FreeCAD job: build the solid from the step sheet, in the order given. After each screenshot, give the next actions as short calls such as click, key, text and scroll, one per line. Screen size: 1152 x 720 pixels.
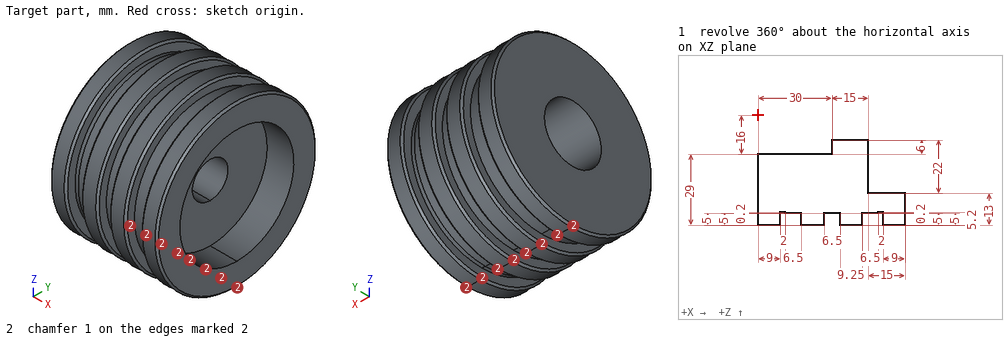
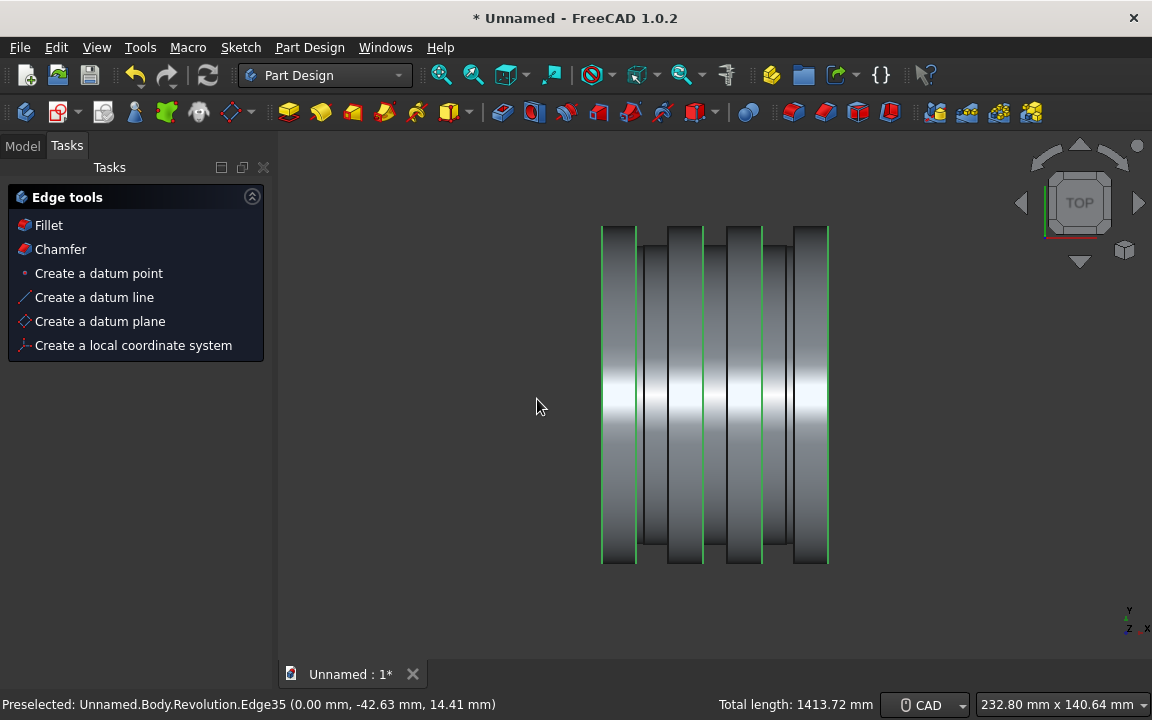
click(794, 394, ctrl)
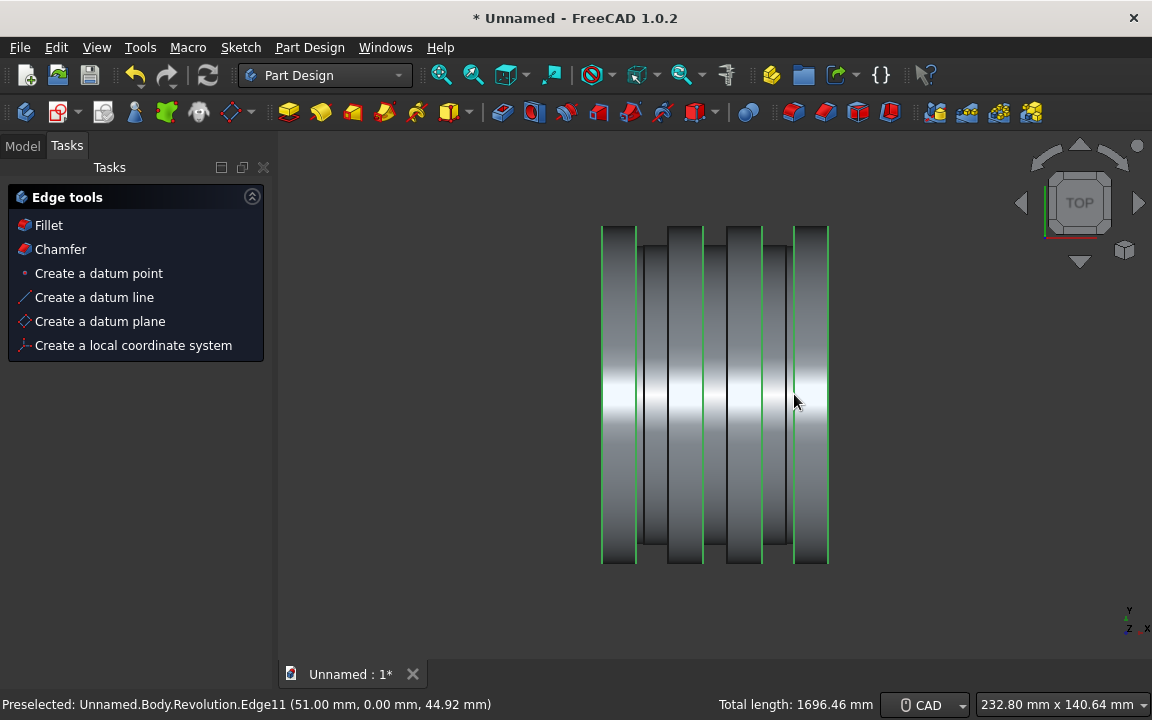
click(727, 394, ctrl)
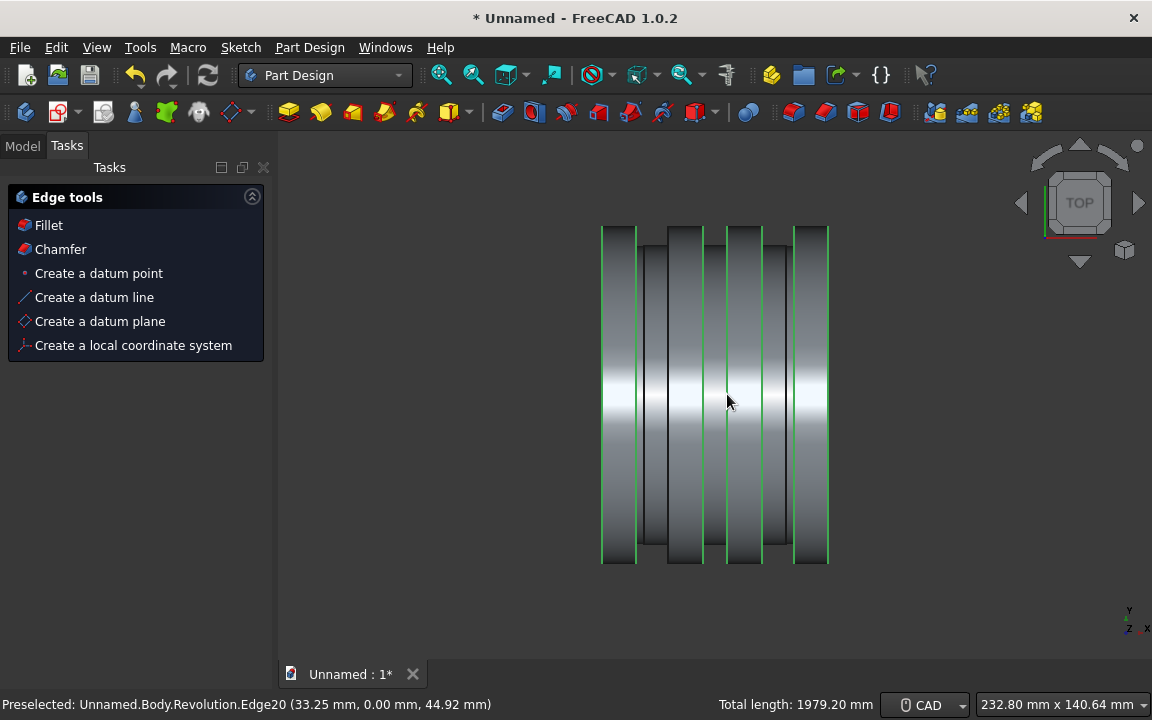
click(668, 394, ctrl)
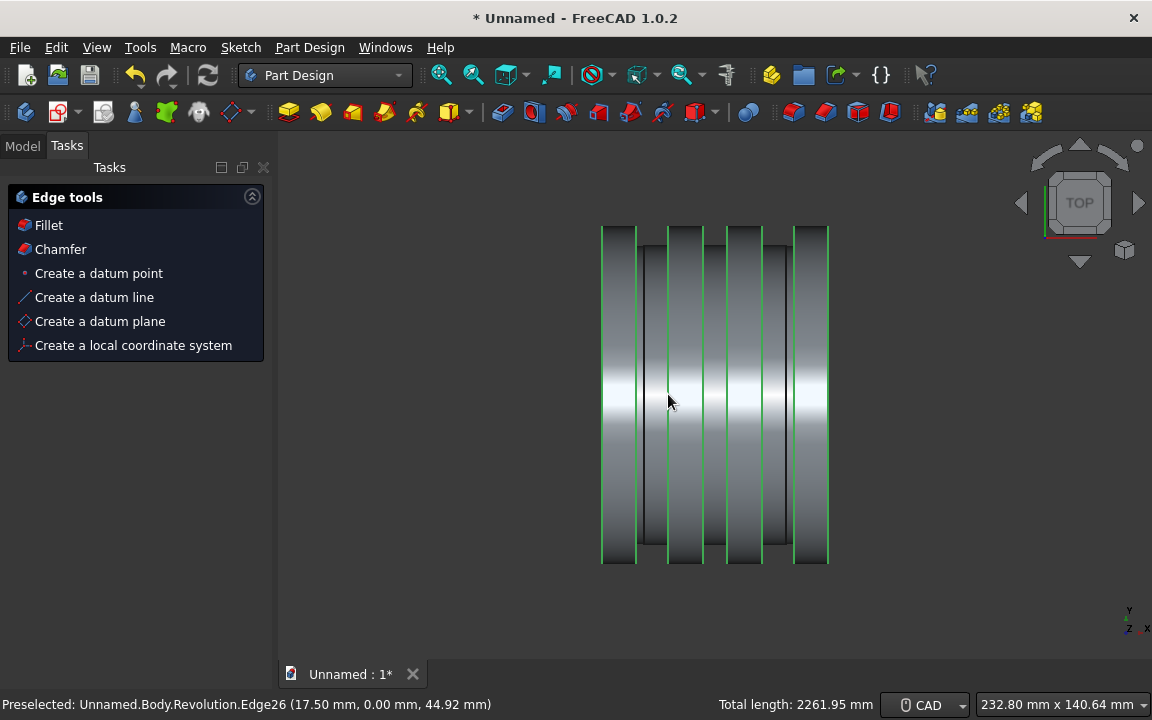
click(826, 112)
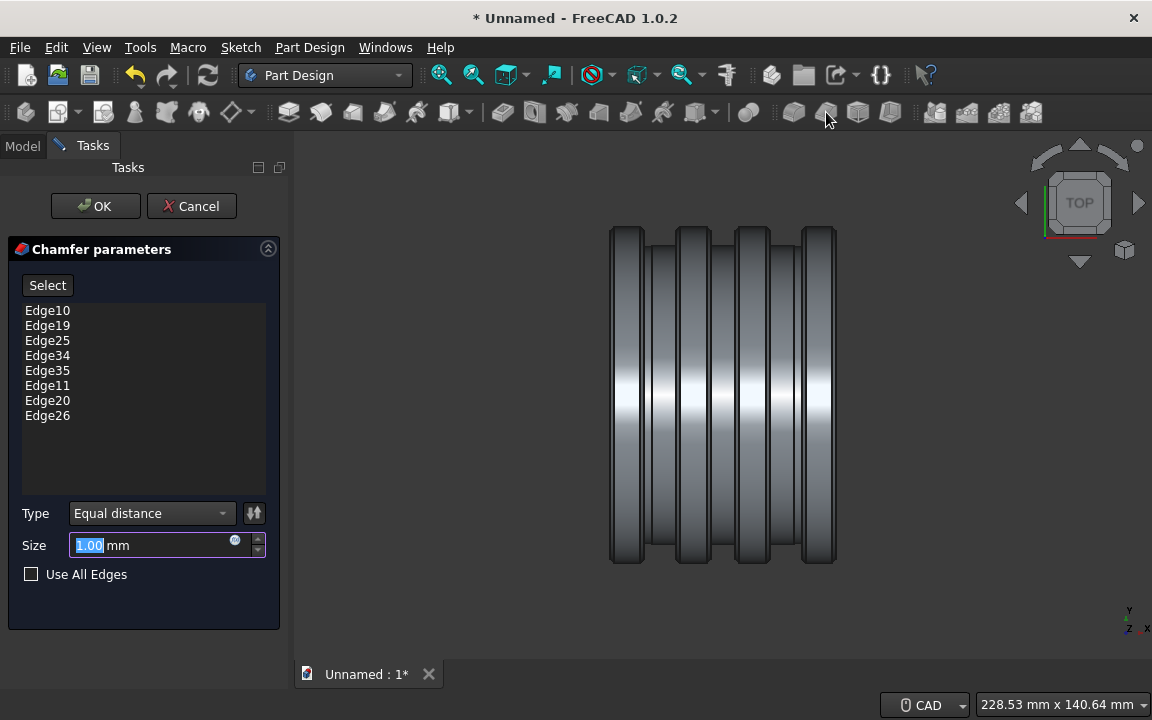
text(1)
key(Tab)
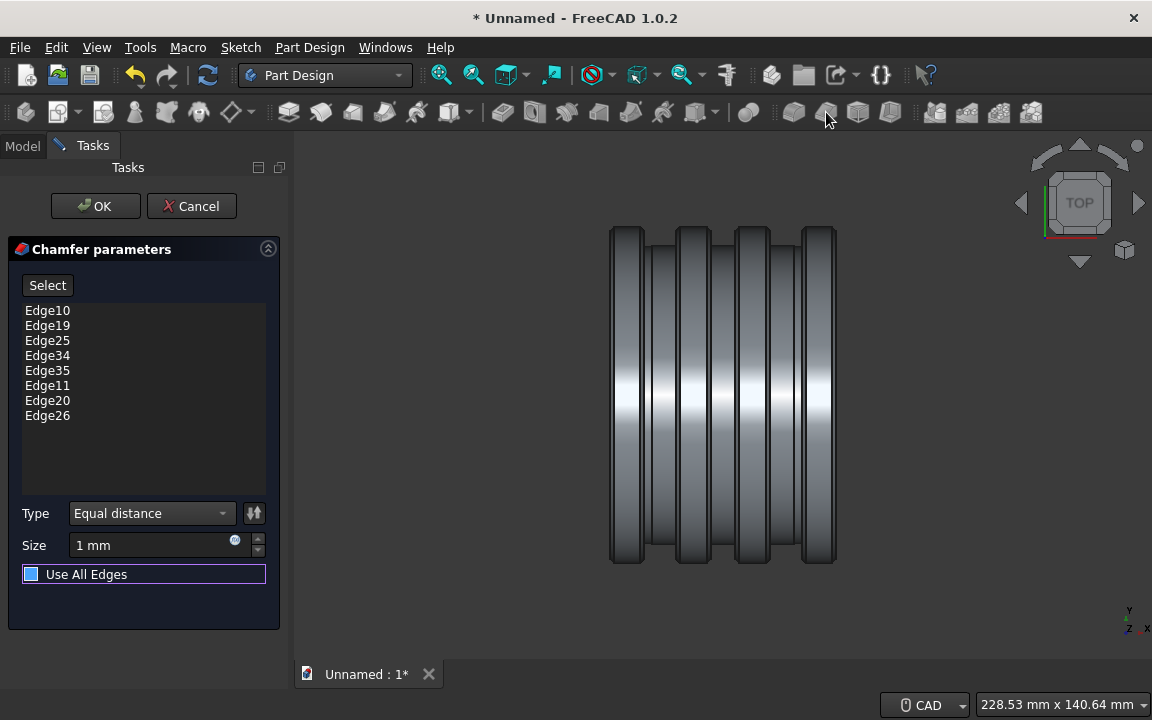
click(96, 206)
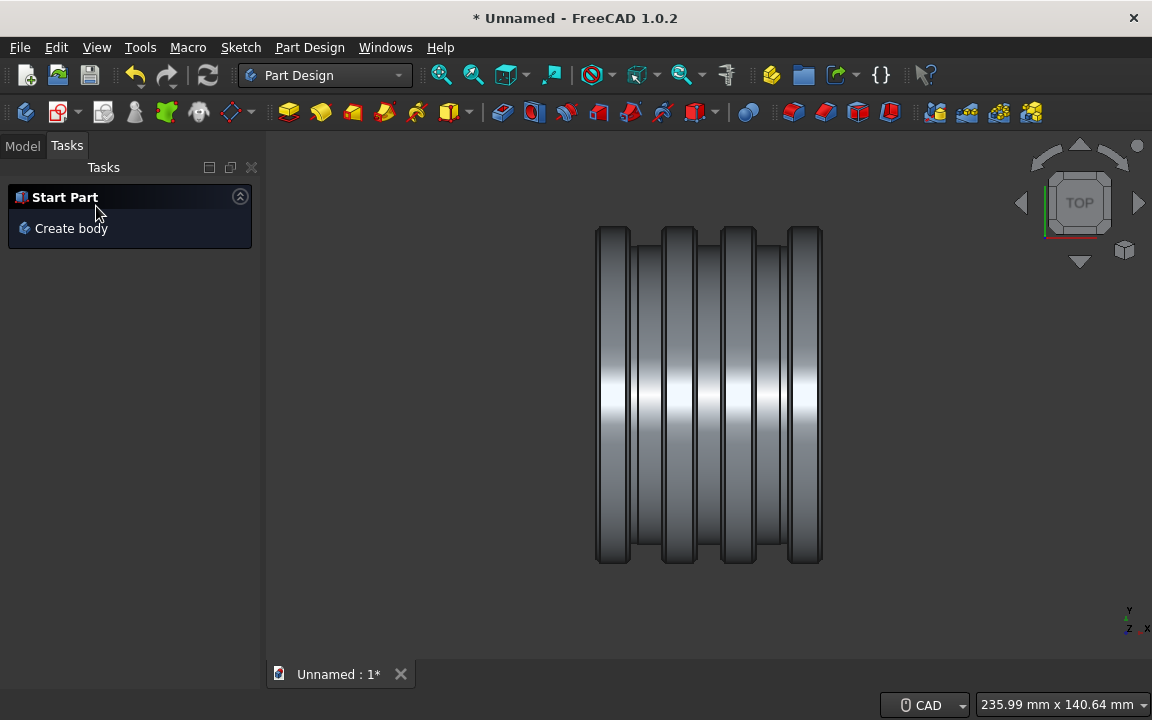
key(0)